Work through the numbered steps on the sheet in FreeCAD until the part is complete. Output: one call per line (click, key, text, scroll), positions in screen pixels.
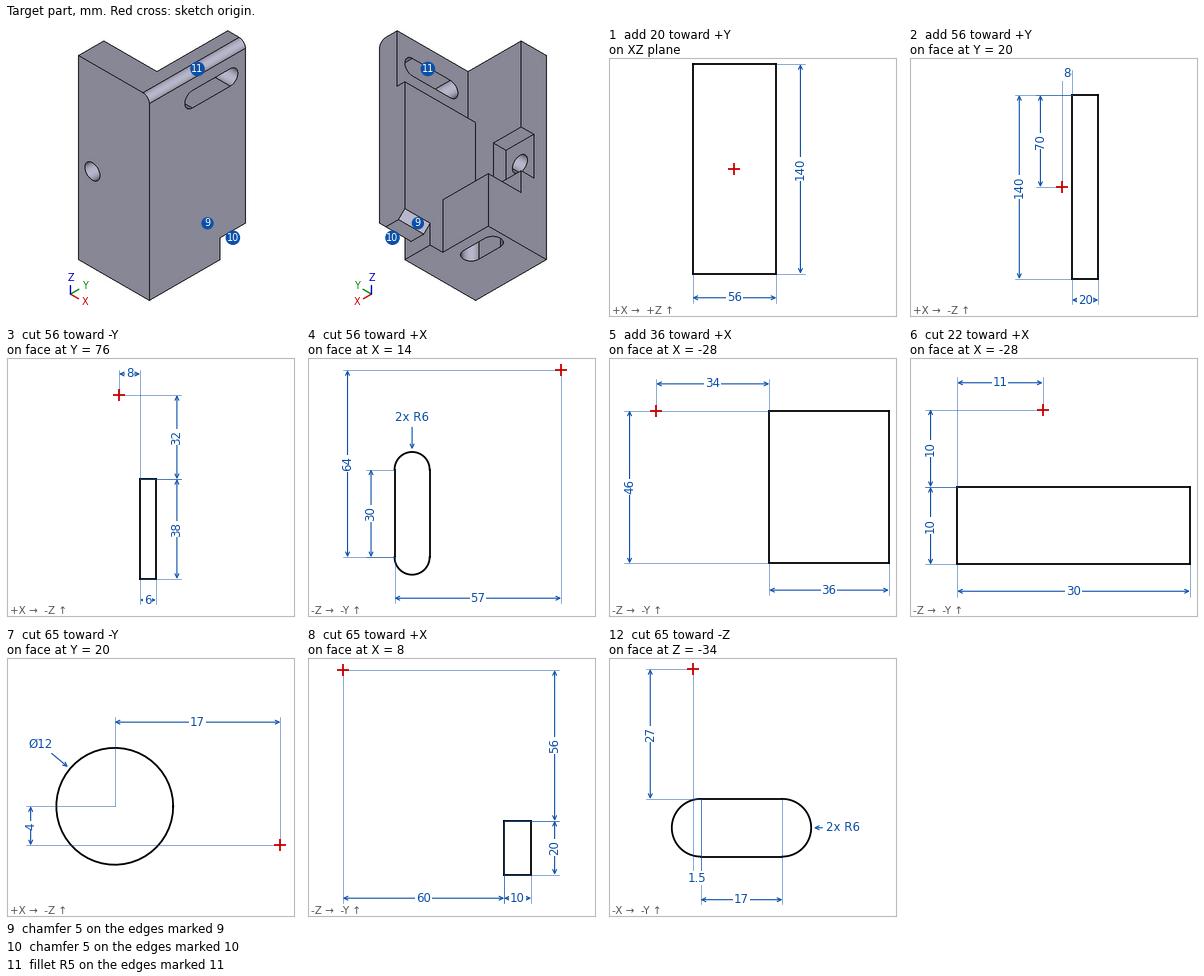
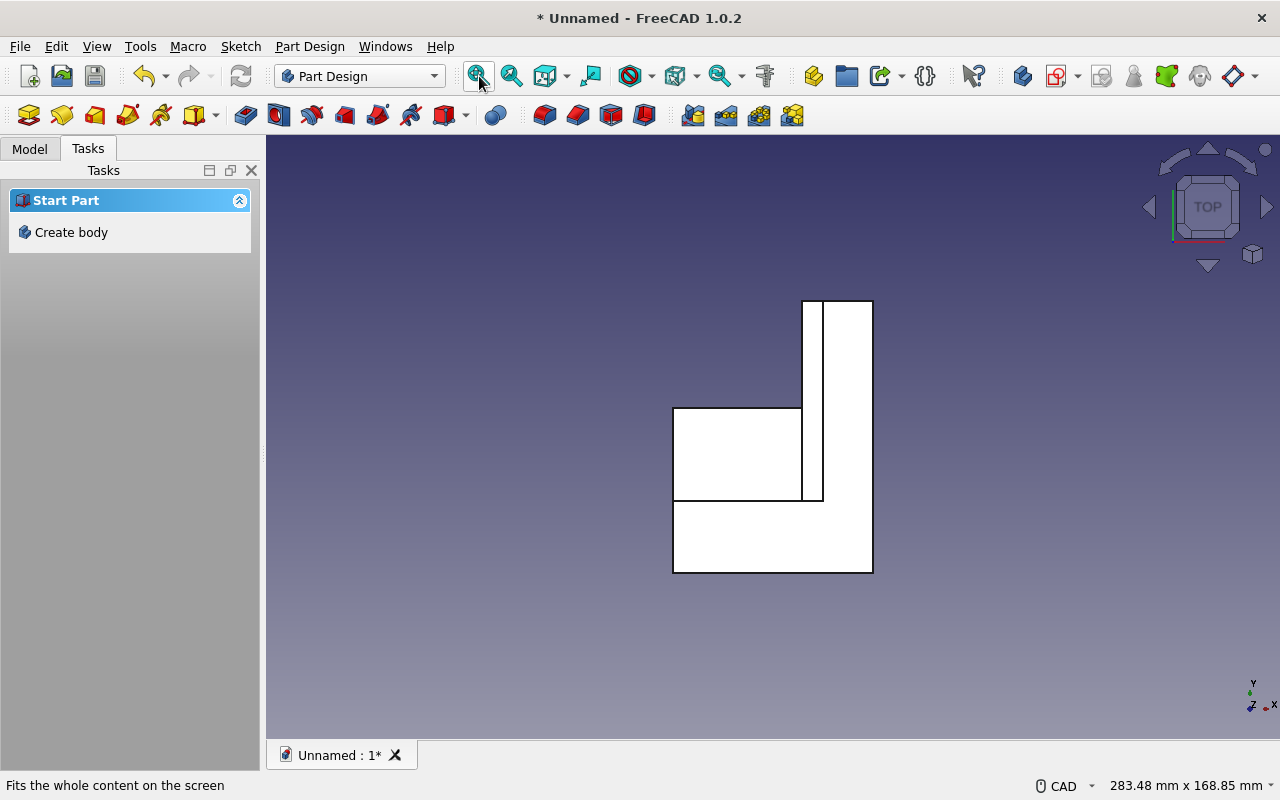
key(1)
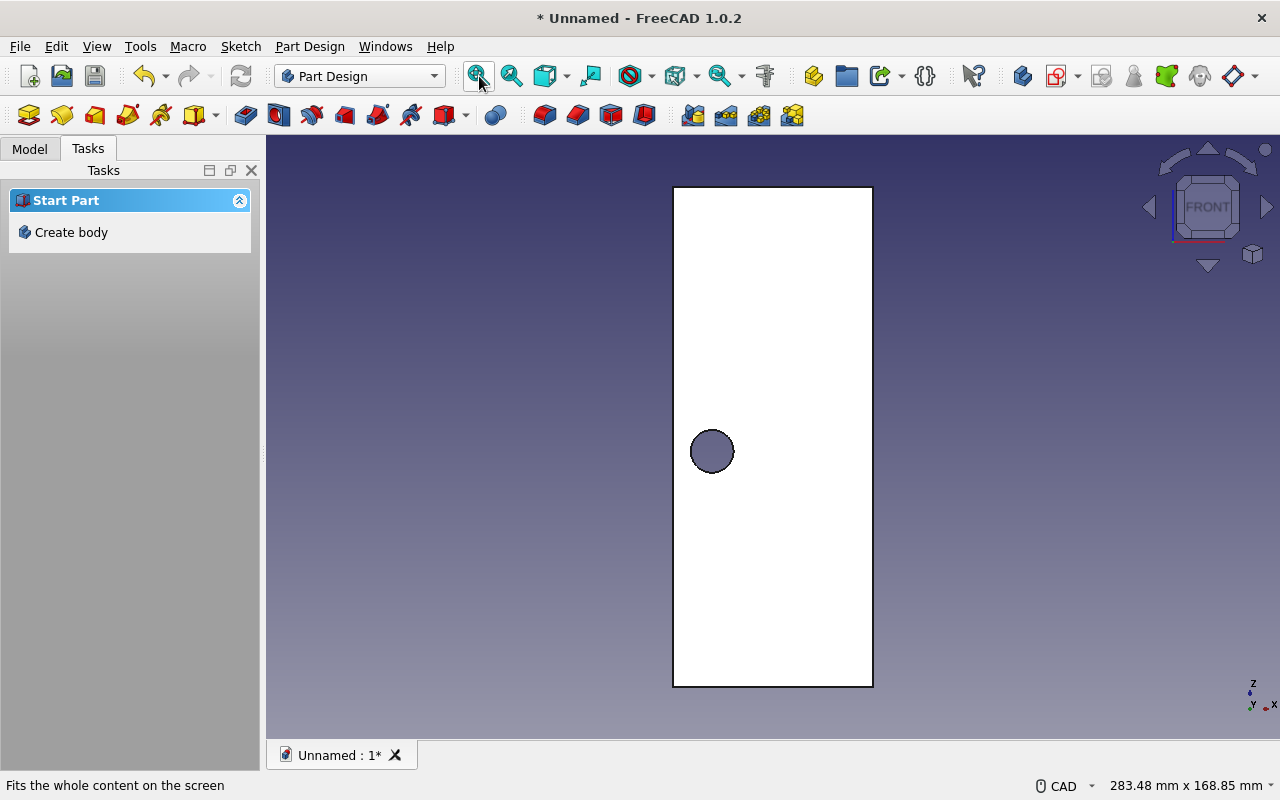
key(3)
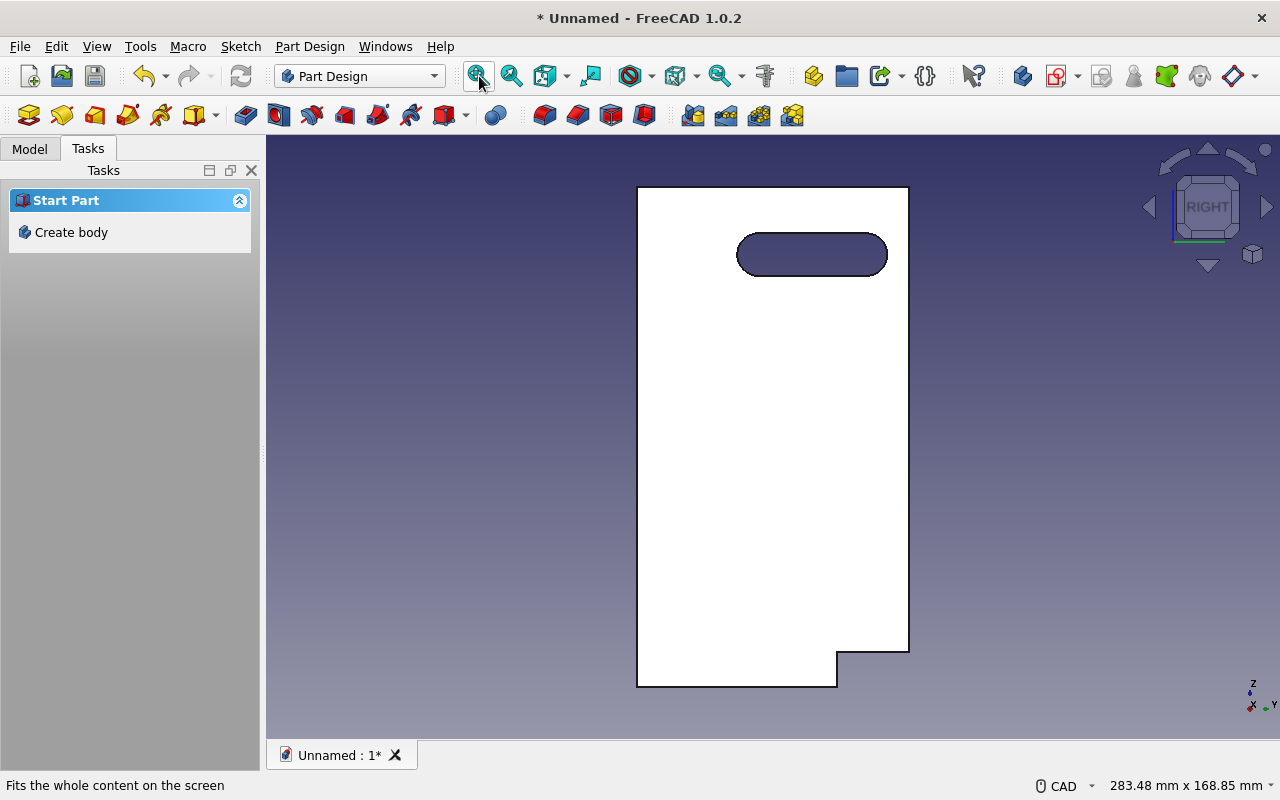
click(873, 651)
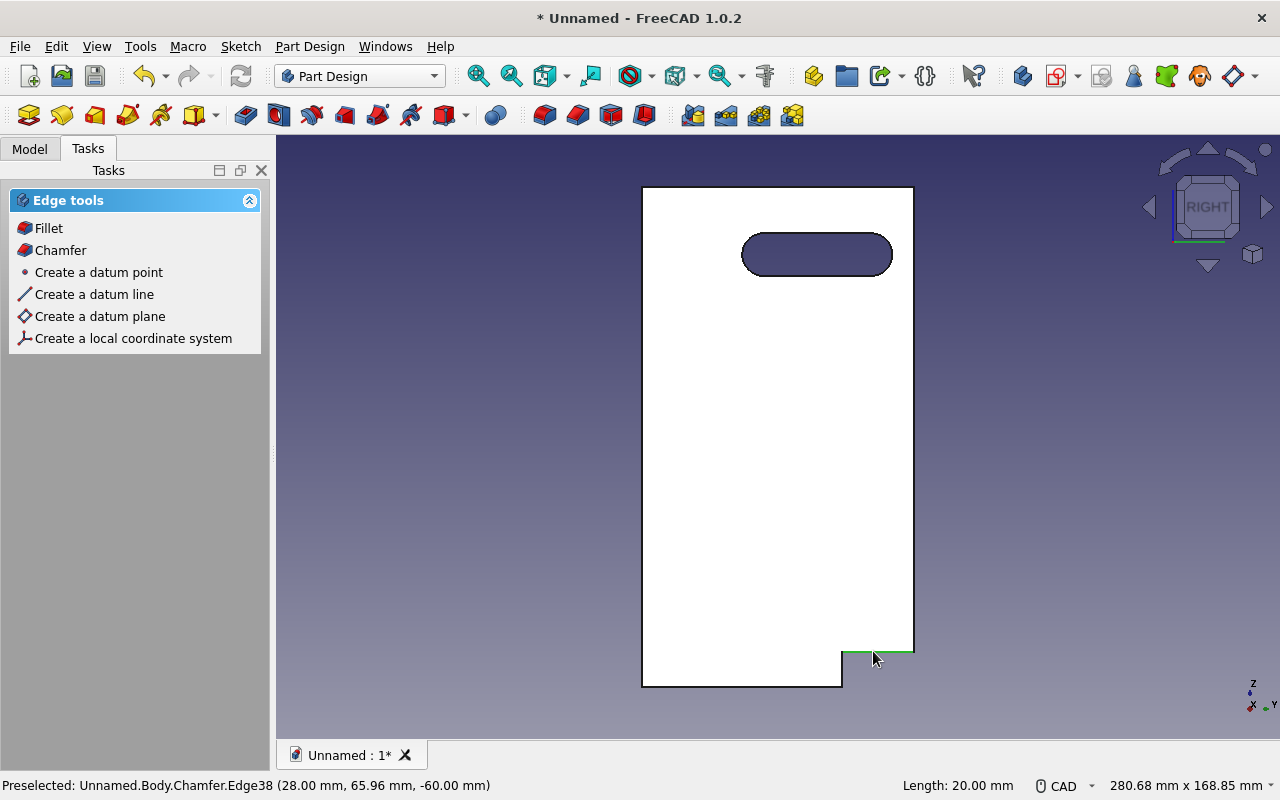
click(578, 116)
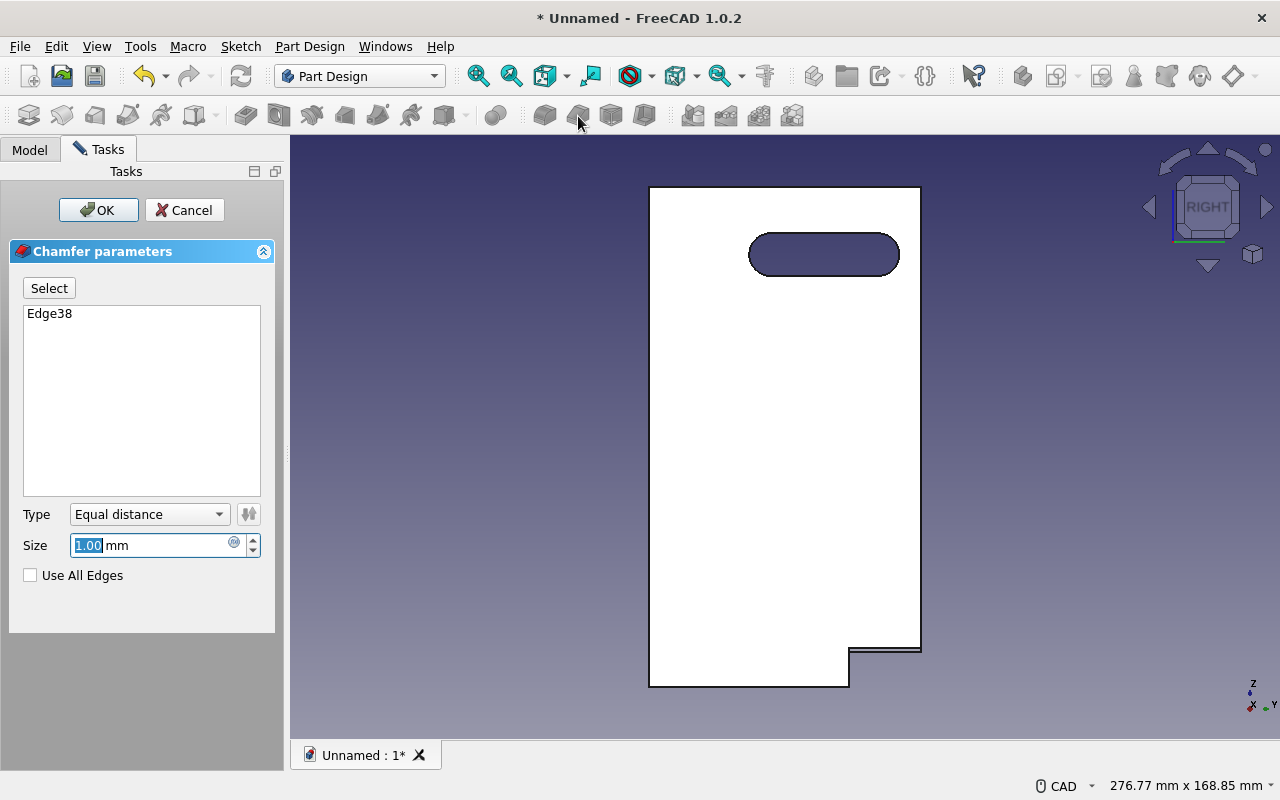
text(5)
key(Tab)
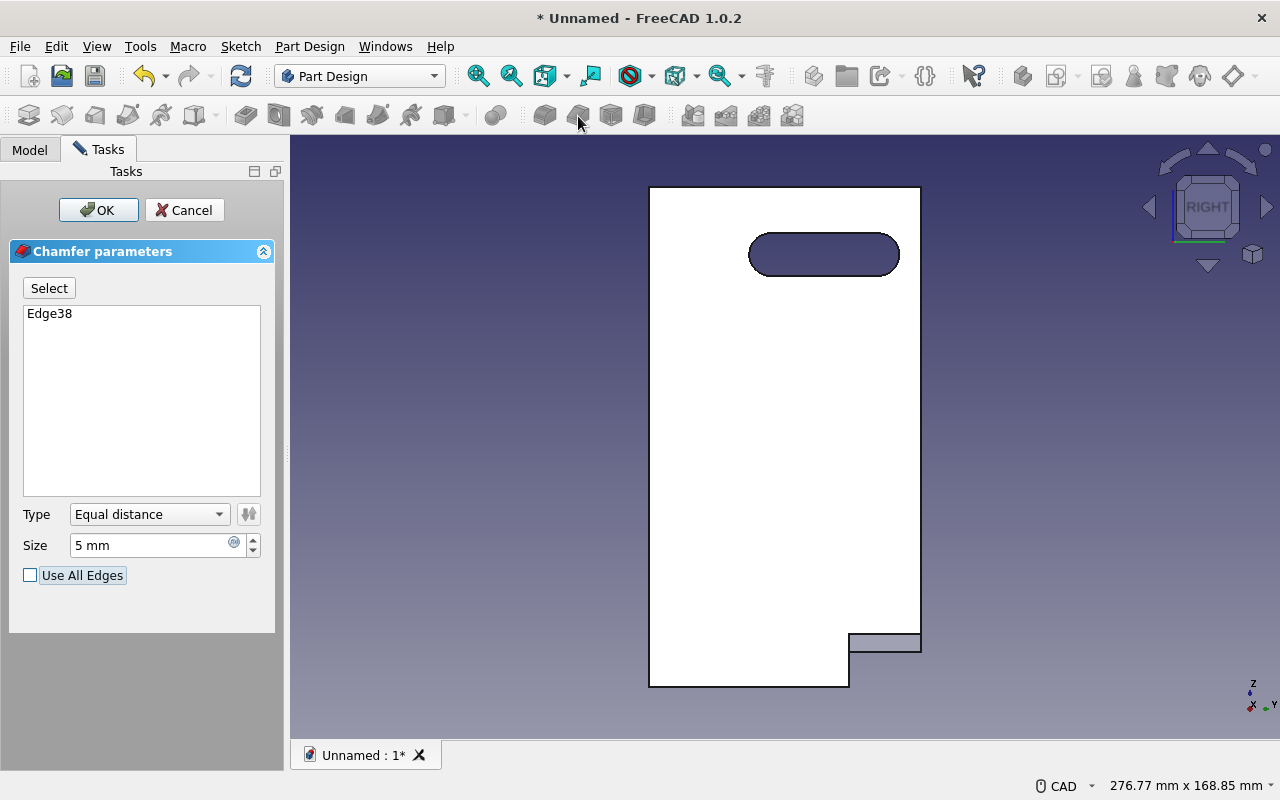
click(99, 210)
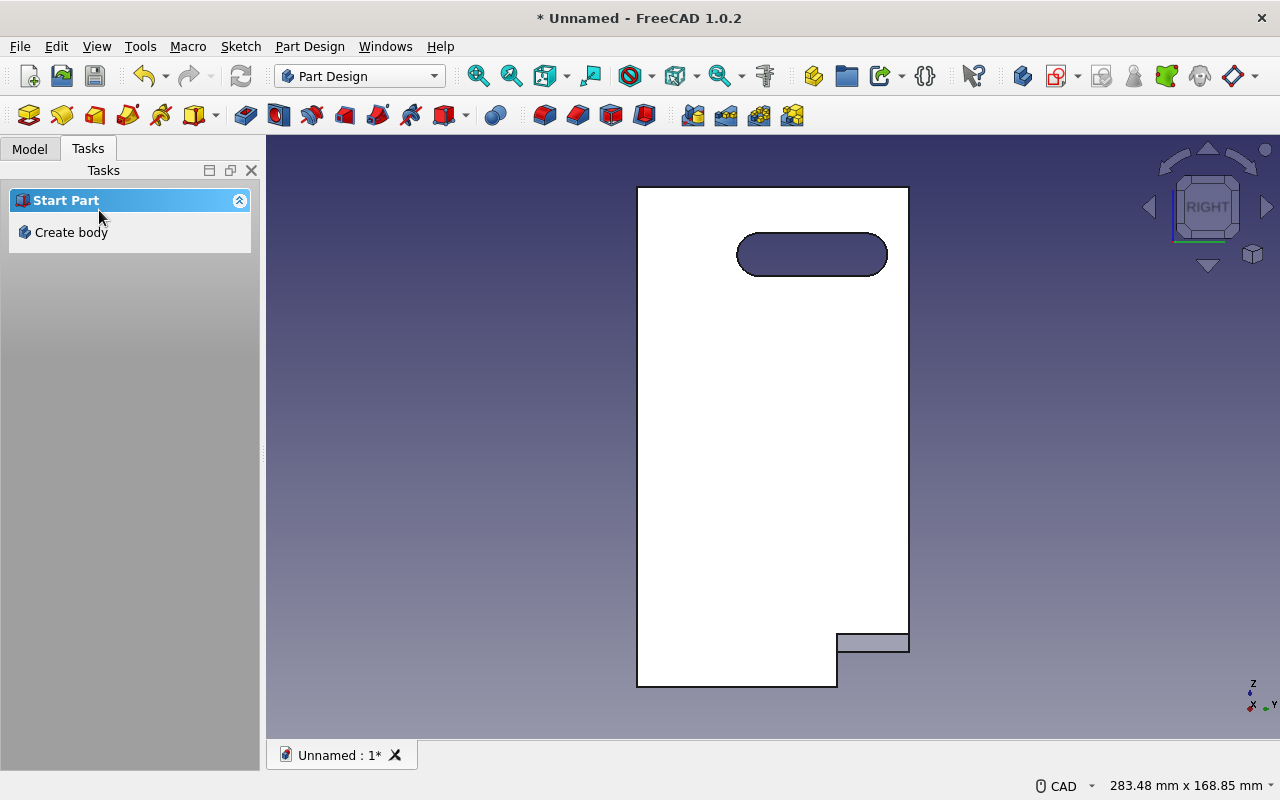
click(773, 186)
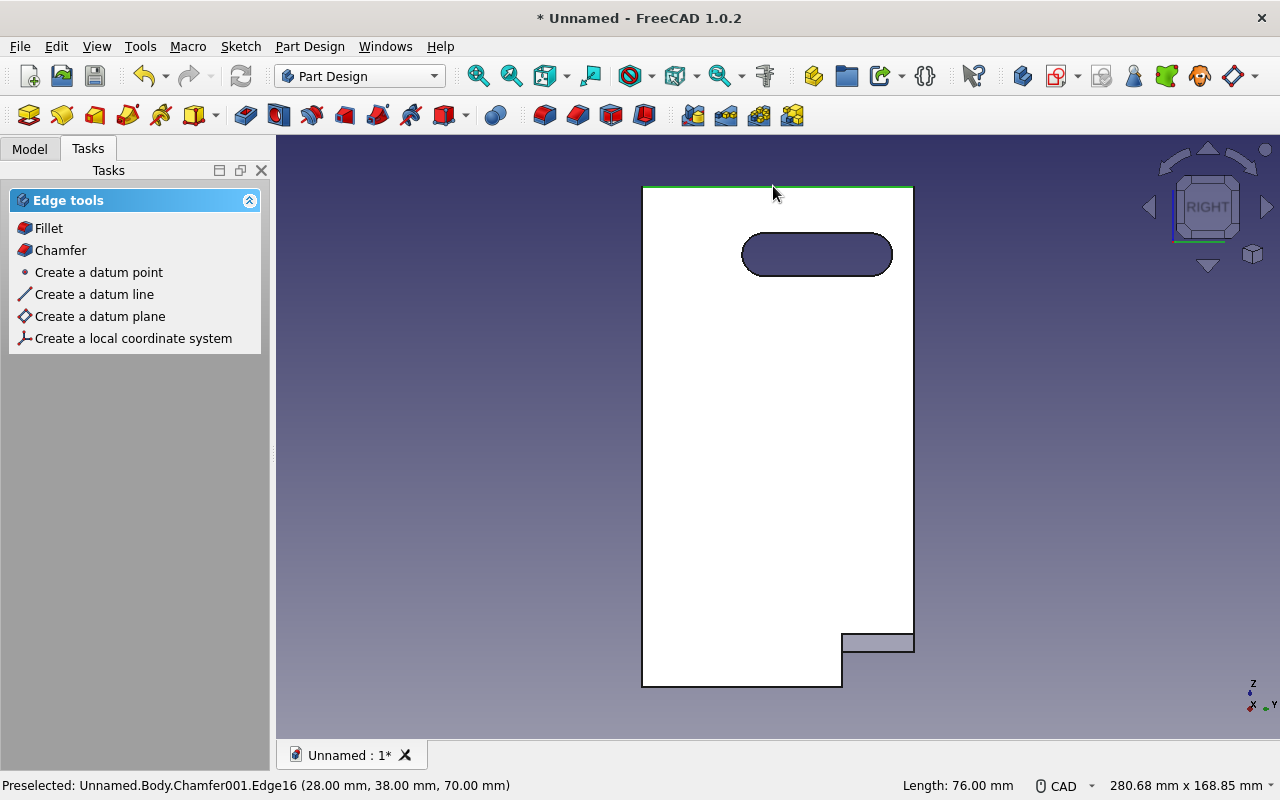
click(545, 116)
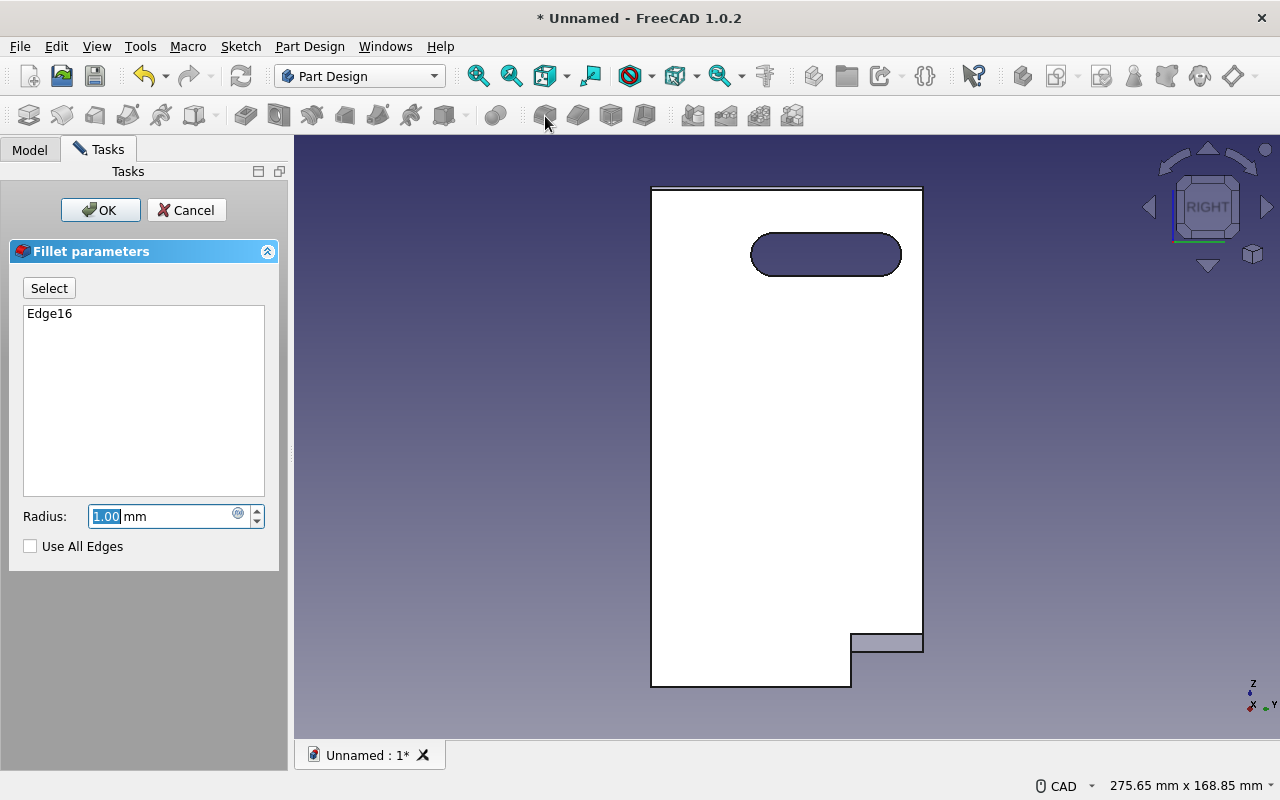
text(5)
key(Tab)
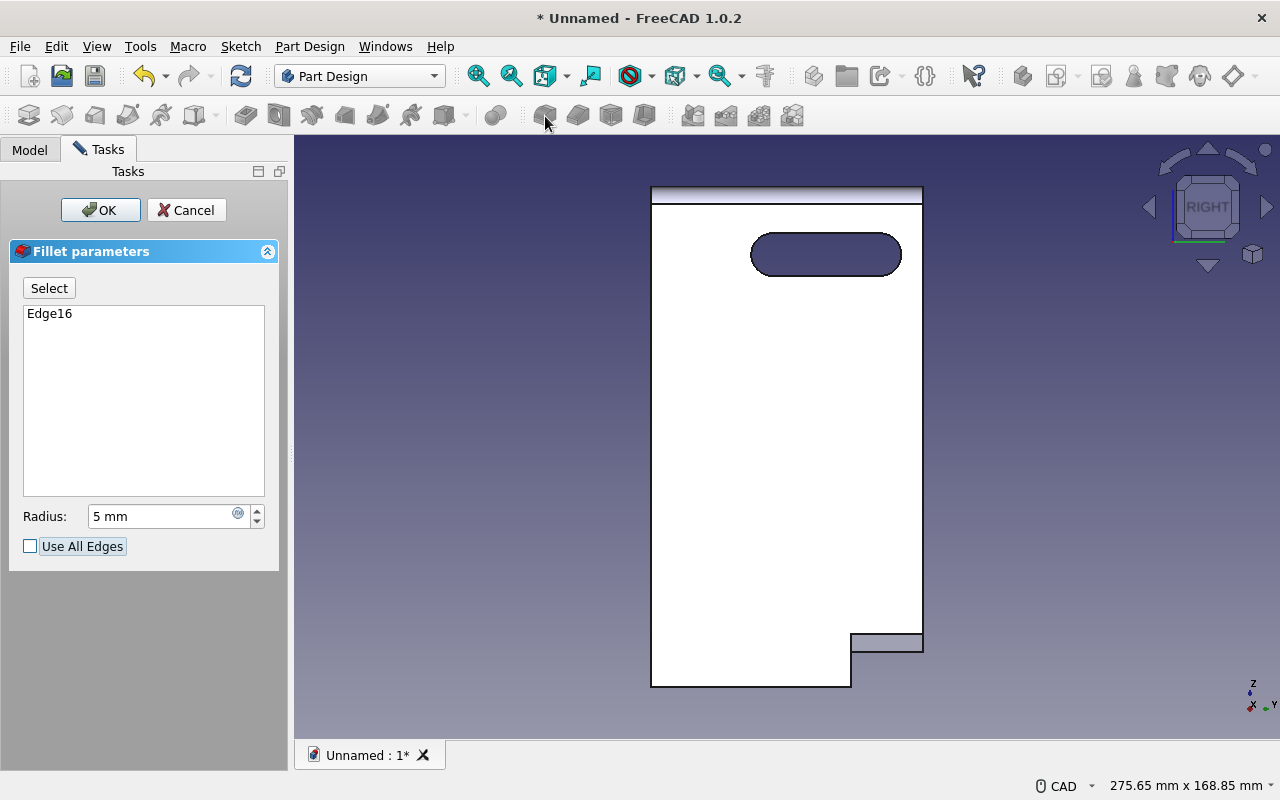
click(101, 210)